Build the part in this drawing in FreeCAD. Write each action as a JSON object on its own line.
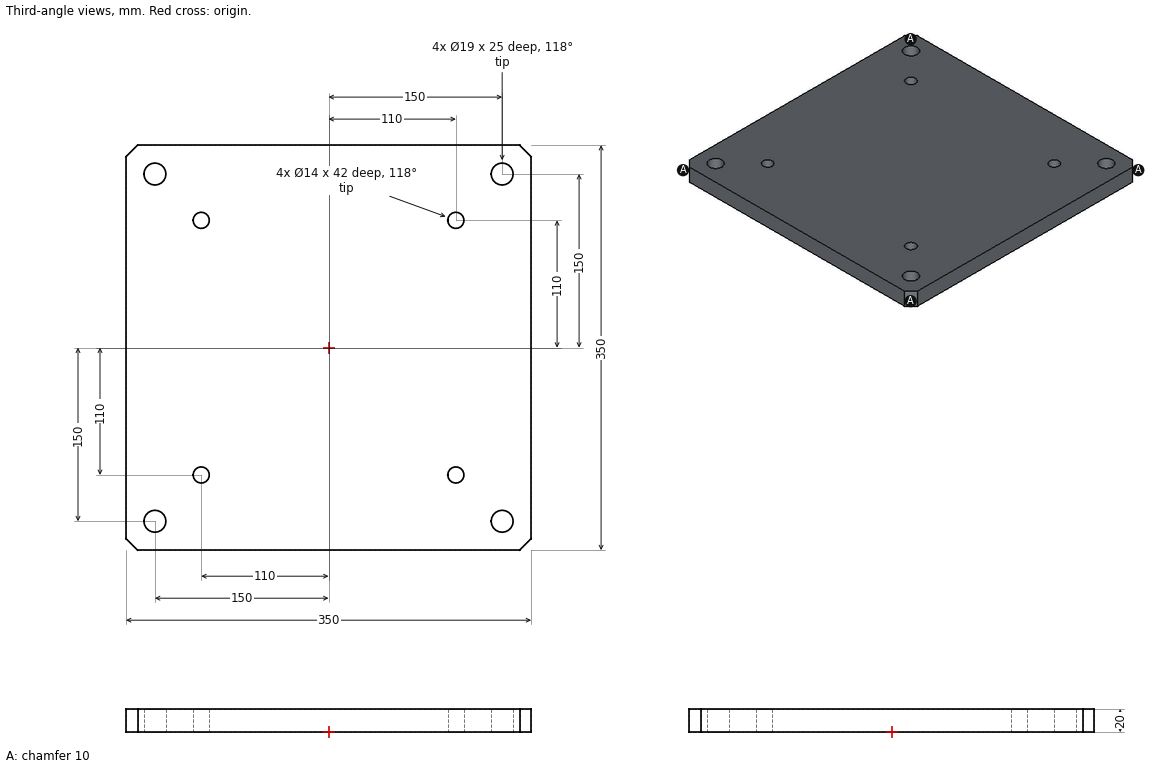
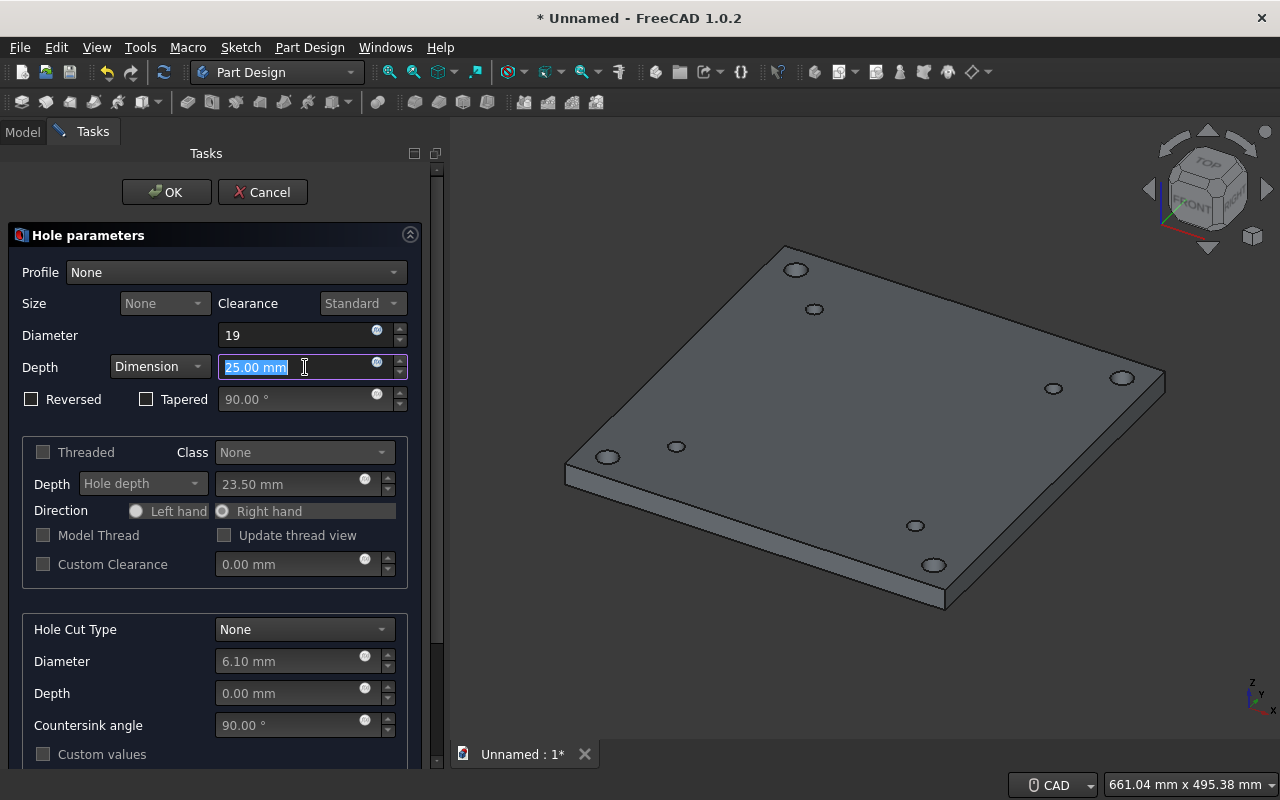
{"action": "type", "text": "25"}
{"action": "key", "text": "Tab"}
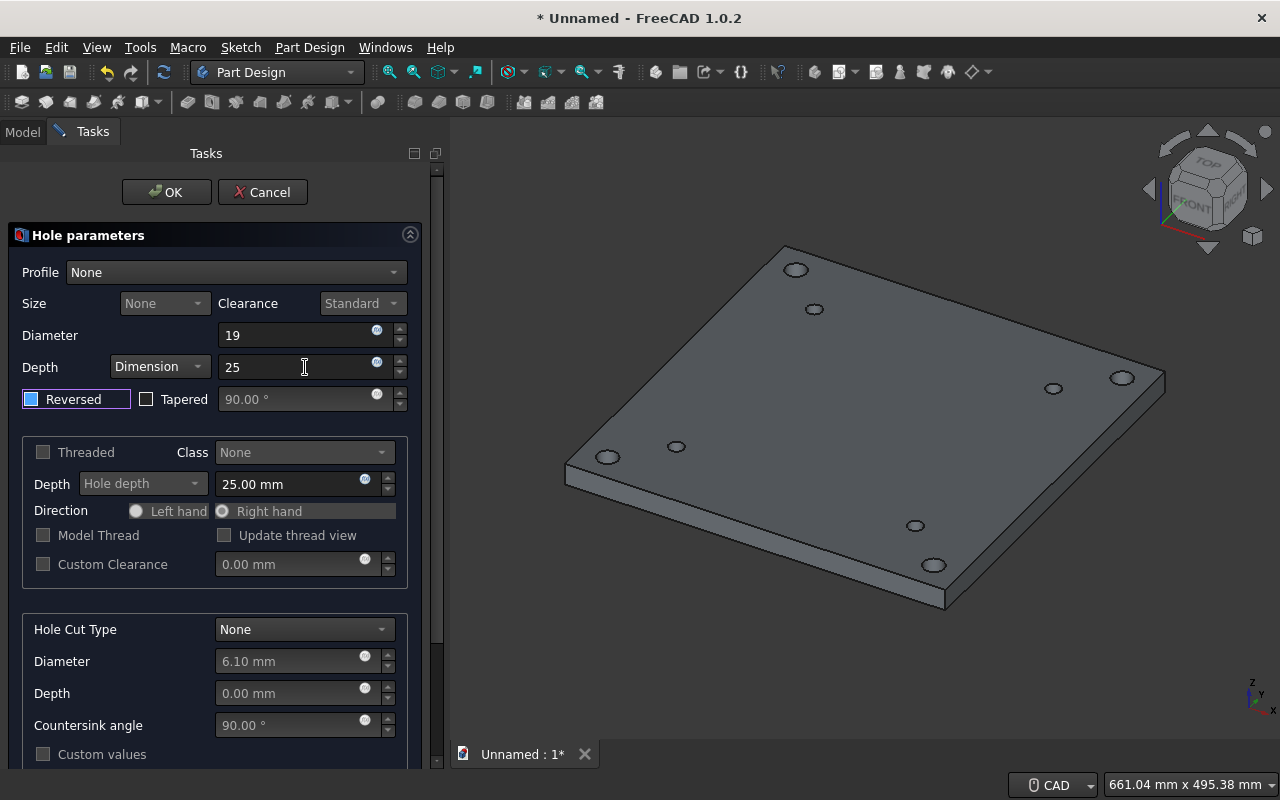
{"action": "left_click", "coordinate": [167, 192]}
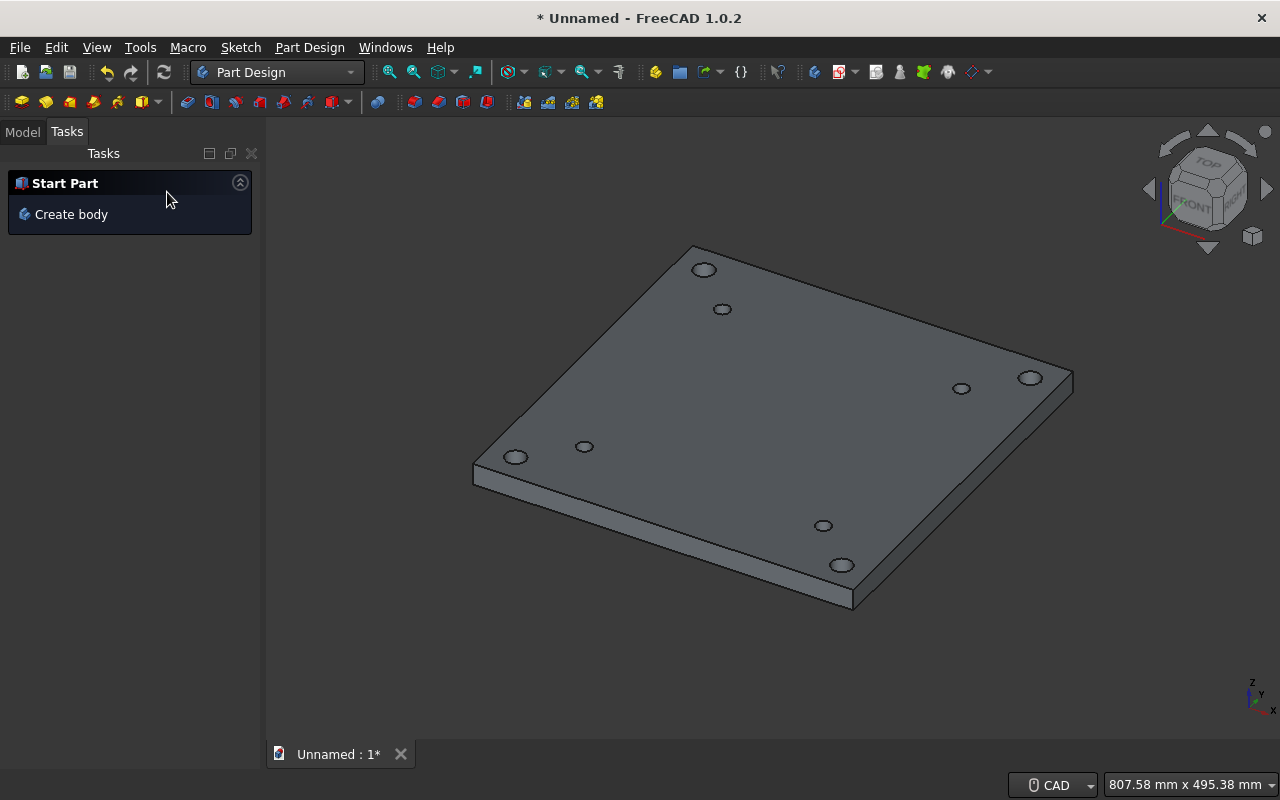
{"action": "left_click", "coordinate": [853, 599]}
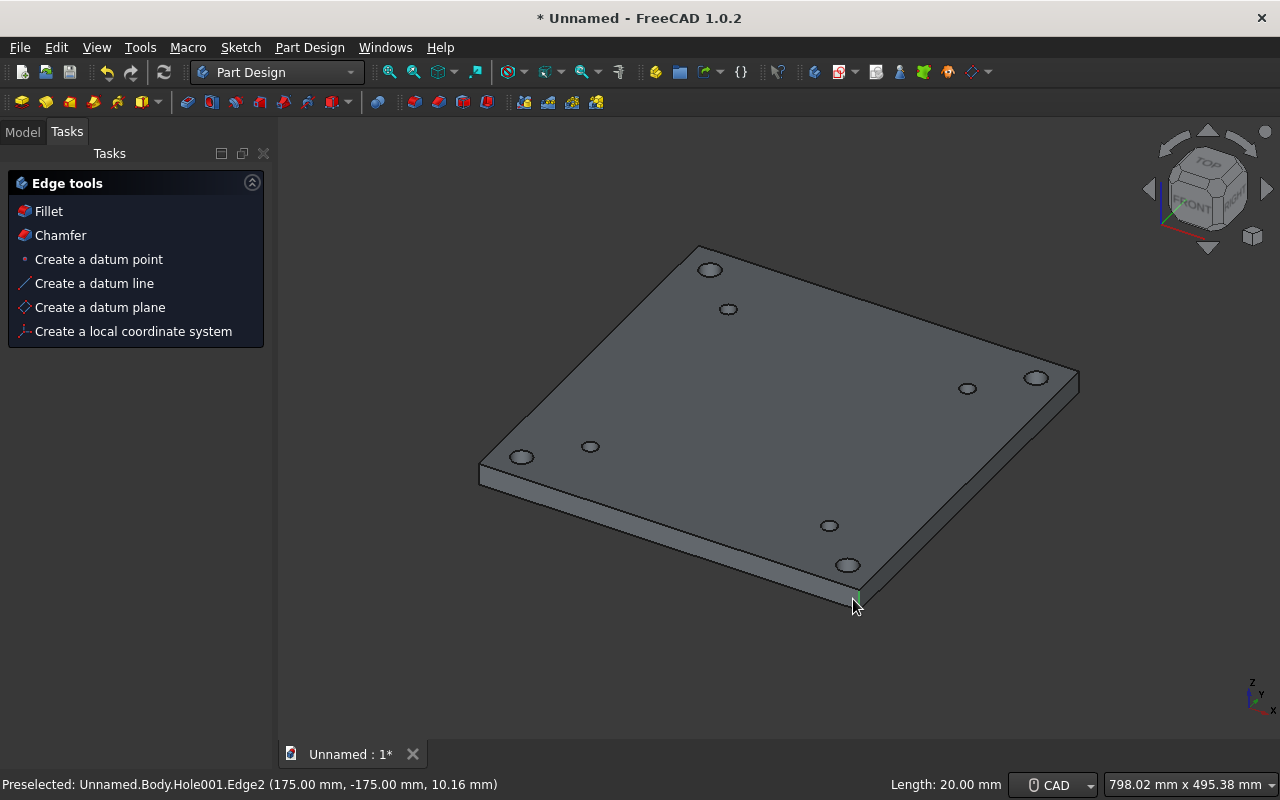
{"action": "key", "text": "0"}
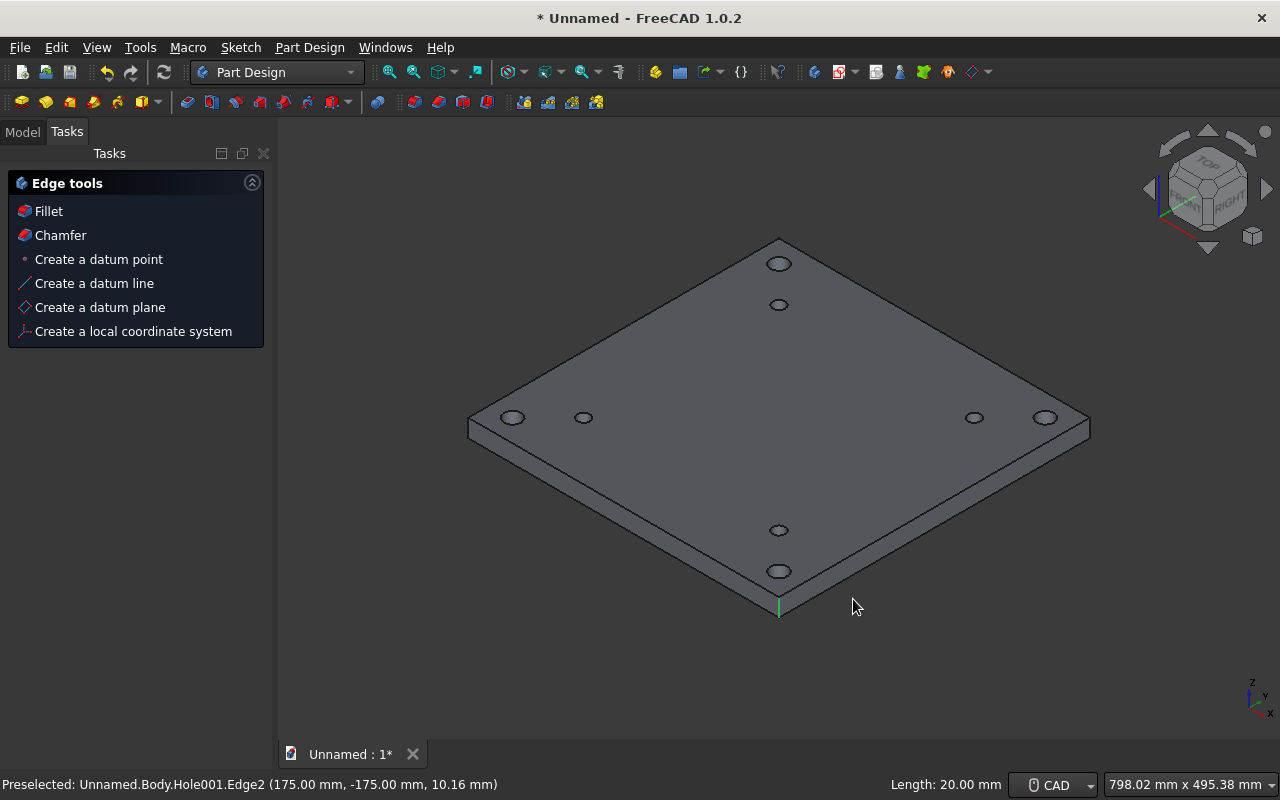
{"action": "key", "text": "2"}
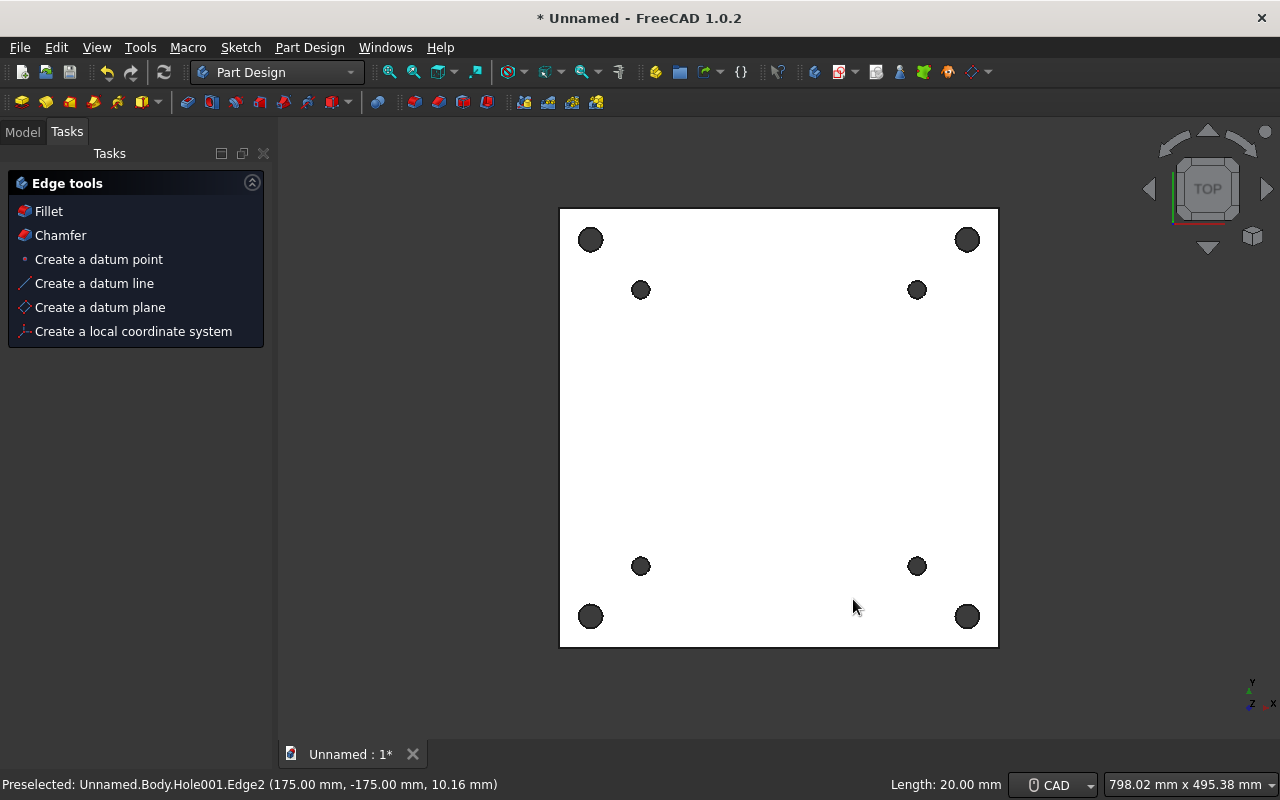
{"action": "key", "text": "1"}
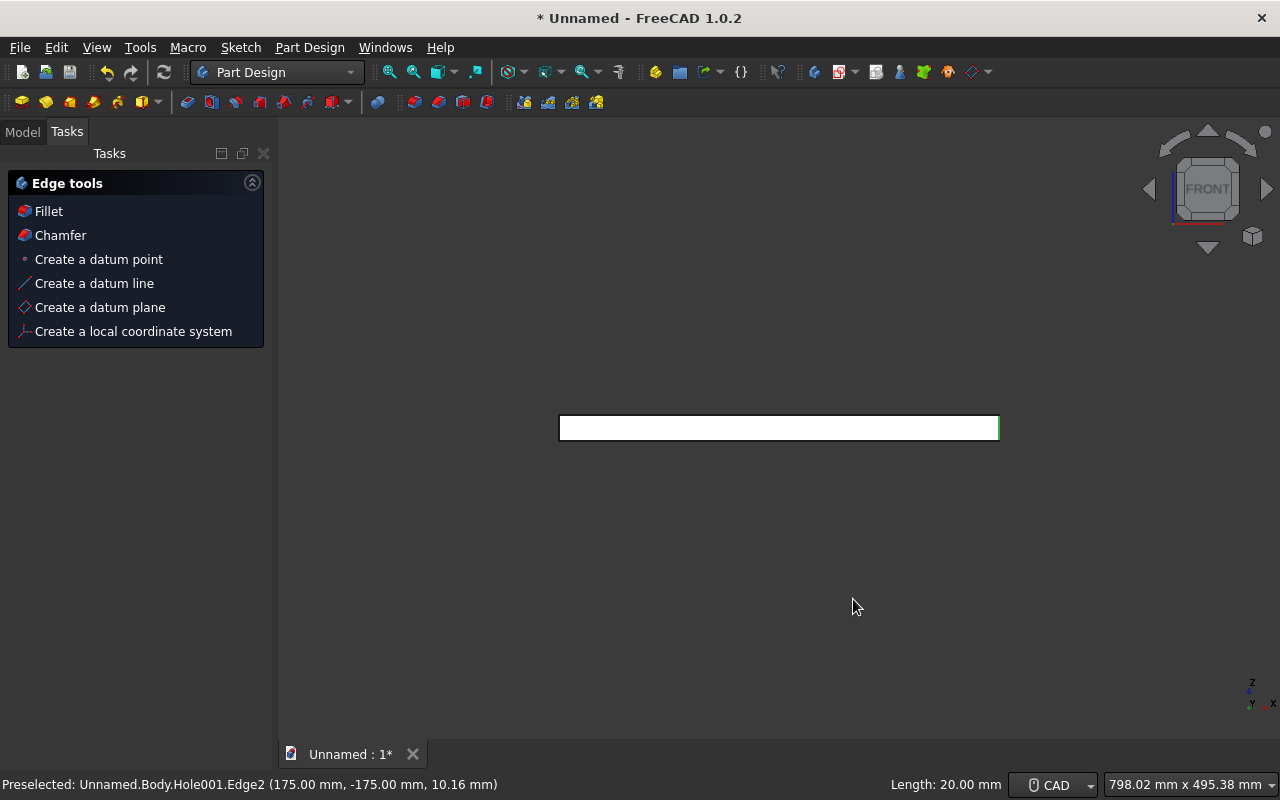
{"action": "left_click", "coordinate": [390, 72]}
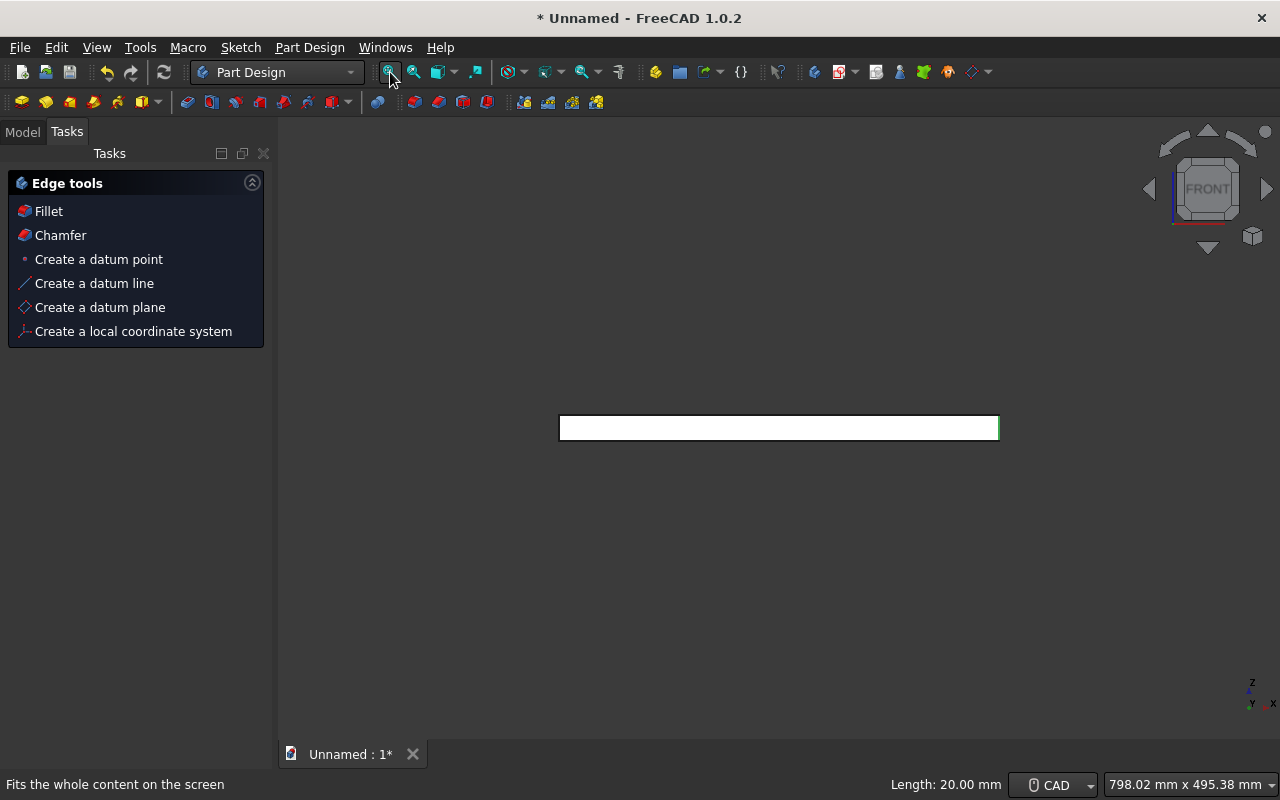
{"action": "left_click", "coordinate": [559, 427], "text": "ctrl"}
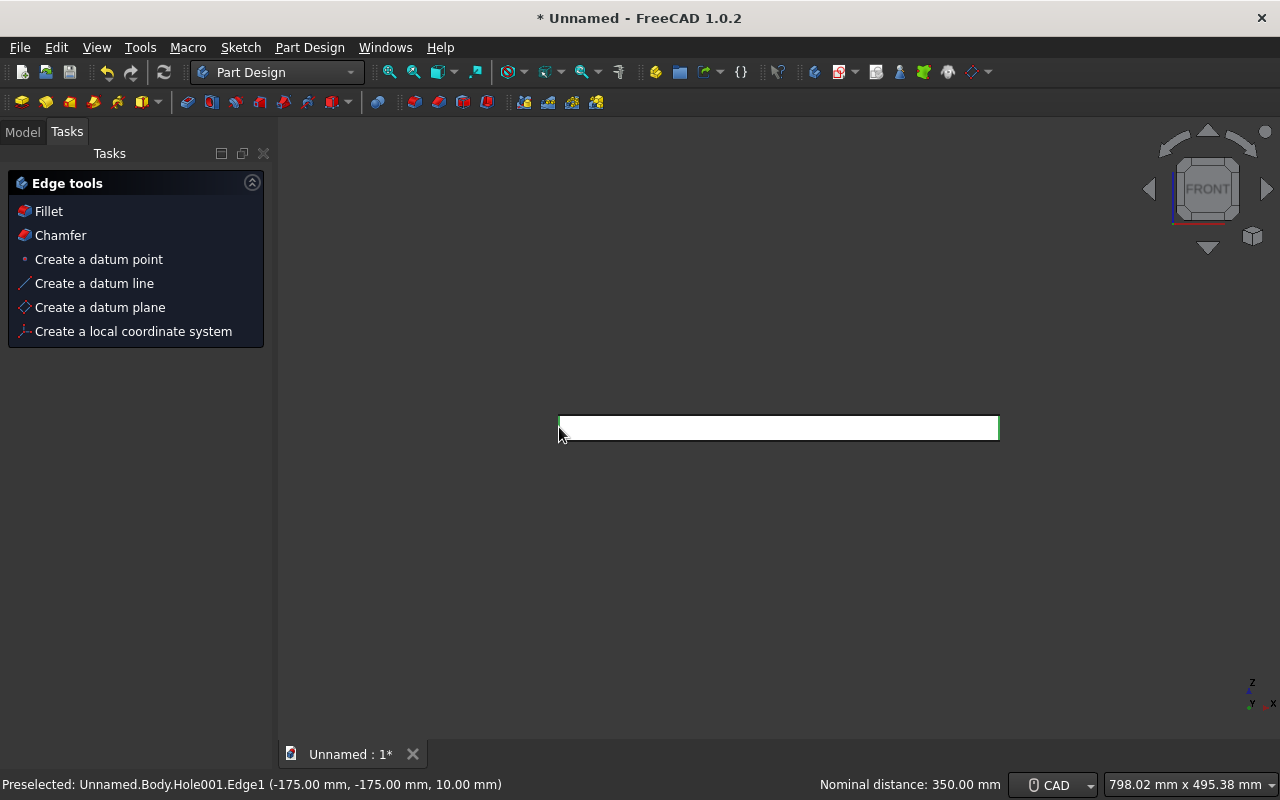
{"action": "key", "text": "3"}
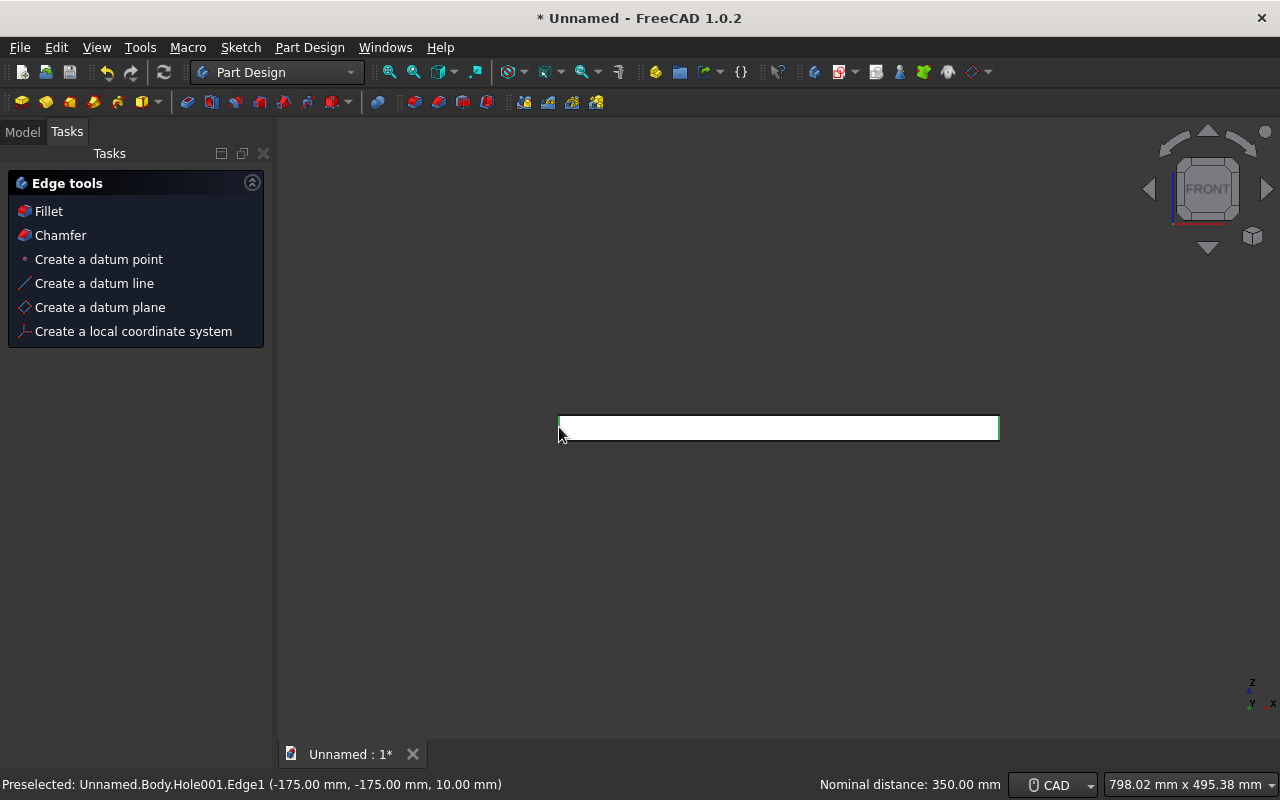
{"action": "left_click", "coordinate": [390, 72]}